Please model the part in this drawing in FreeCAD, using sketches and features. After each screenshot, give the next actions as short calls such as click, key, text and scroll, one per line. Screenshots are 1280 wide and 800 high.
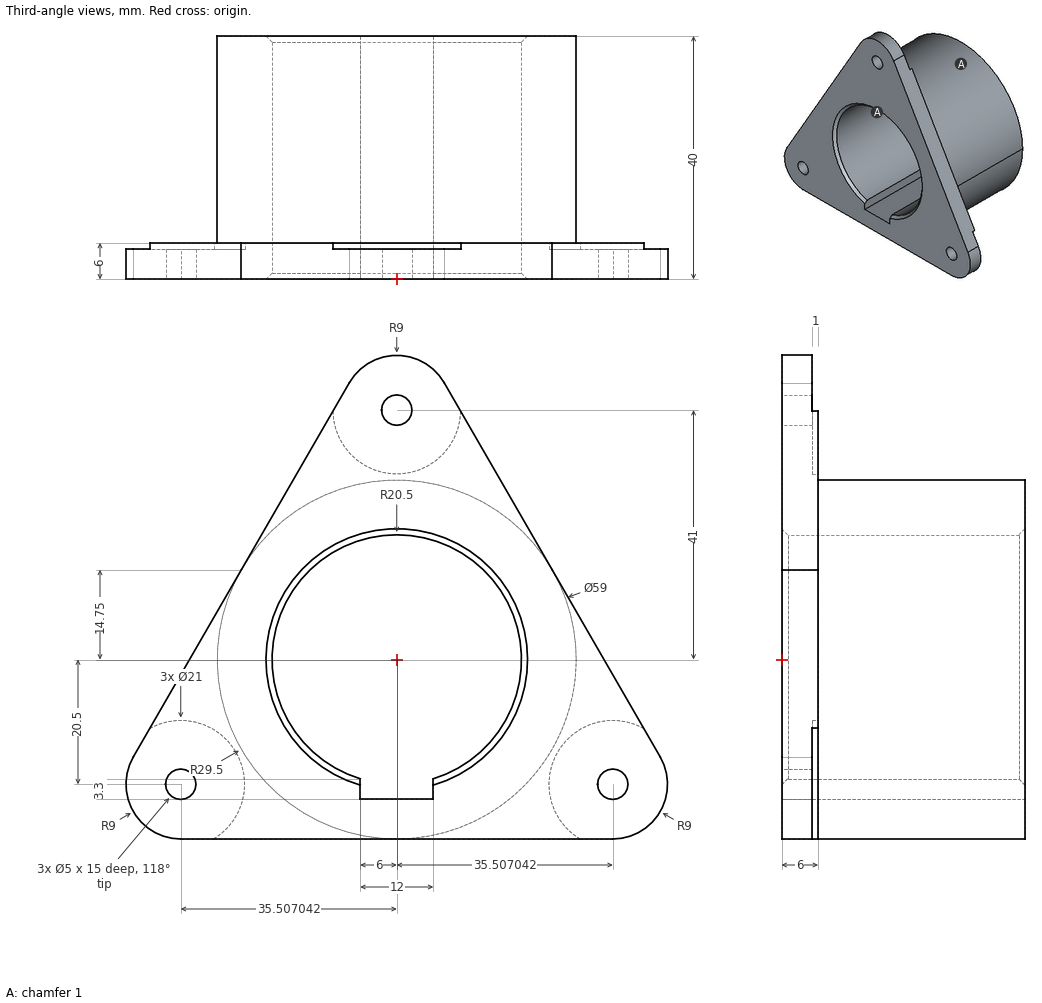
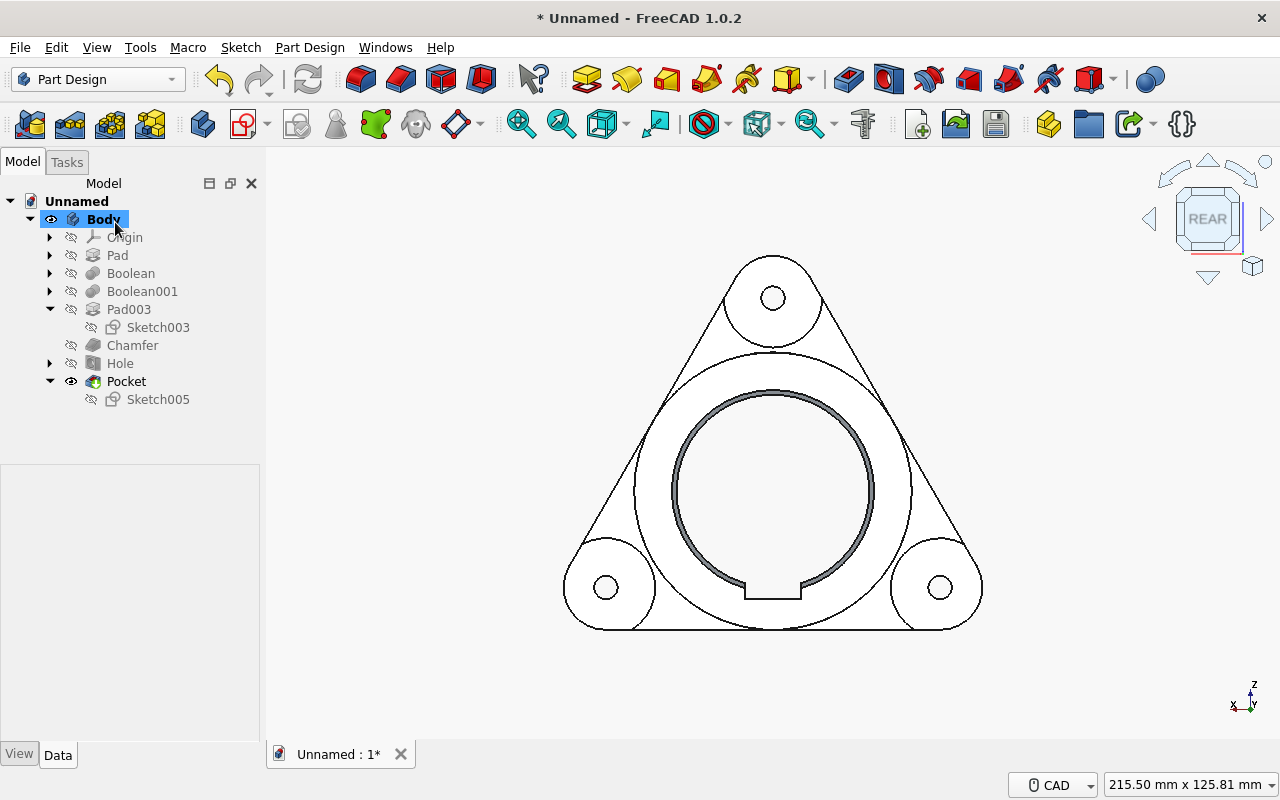
key(0)